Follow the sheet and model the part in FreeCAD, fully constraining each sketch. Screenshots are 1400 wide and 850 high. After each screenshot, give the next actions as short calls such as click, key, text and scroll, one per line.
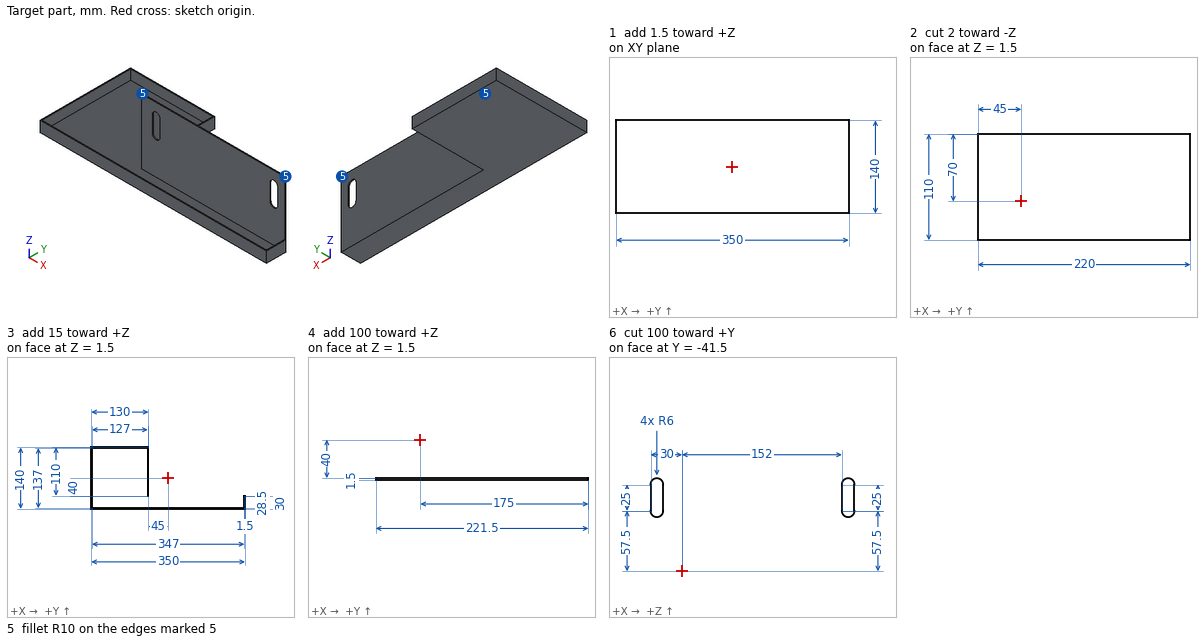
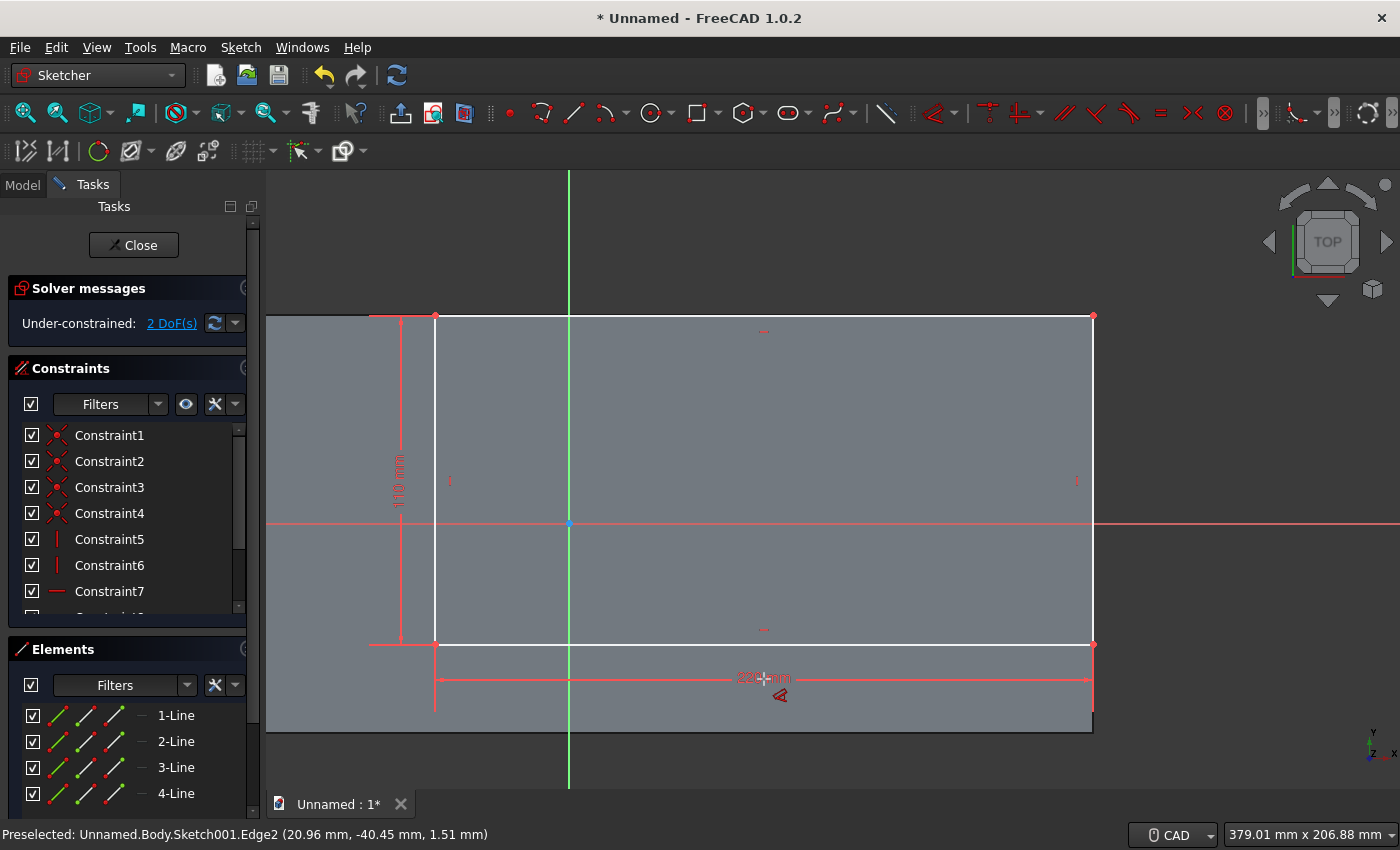
click(435, 316)
click(502, 282)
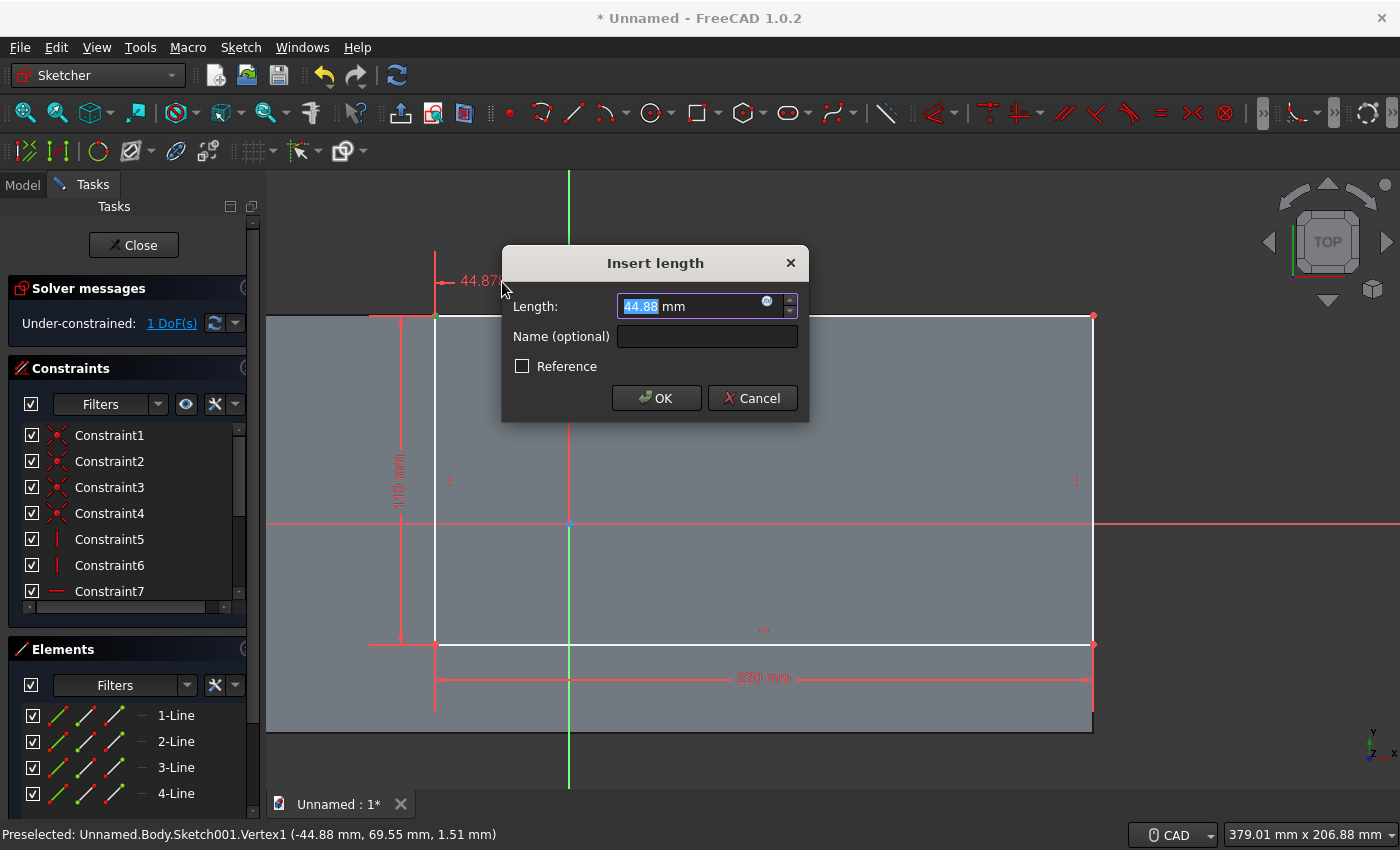
text(45)
key(Return)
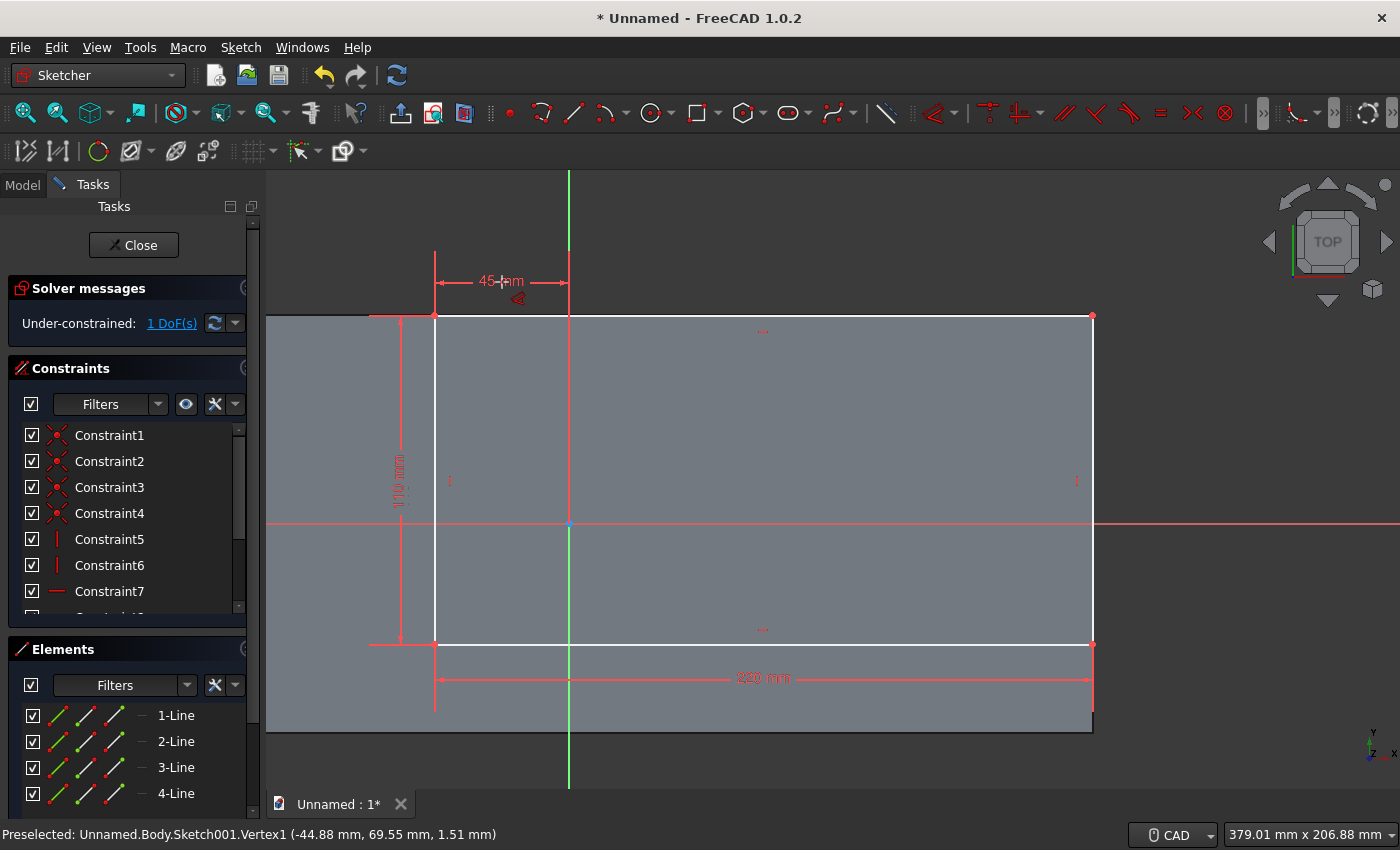
click(435, 316)
click(401, 420)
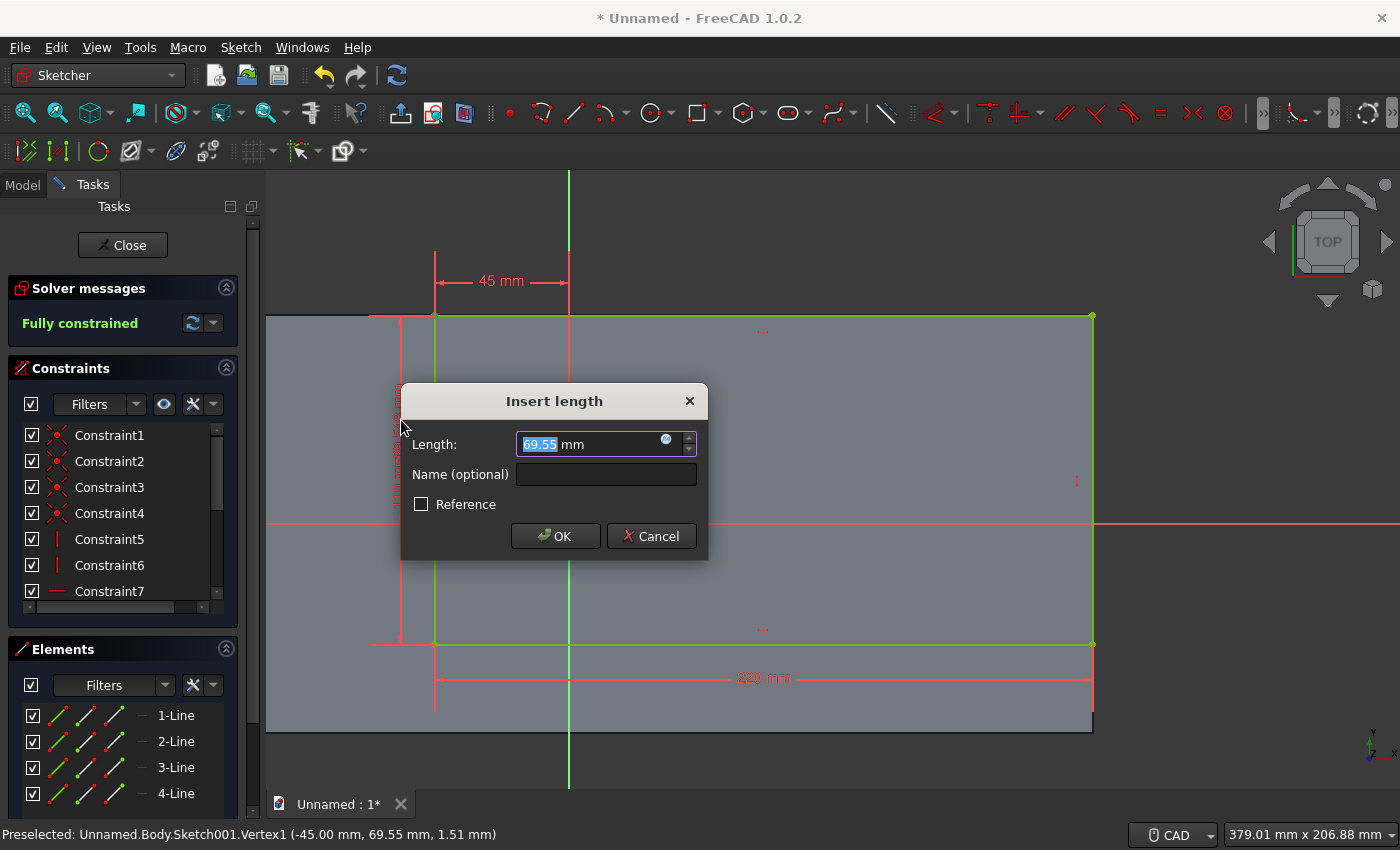
text(70)
key(Return)
key(Escape)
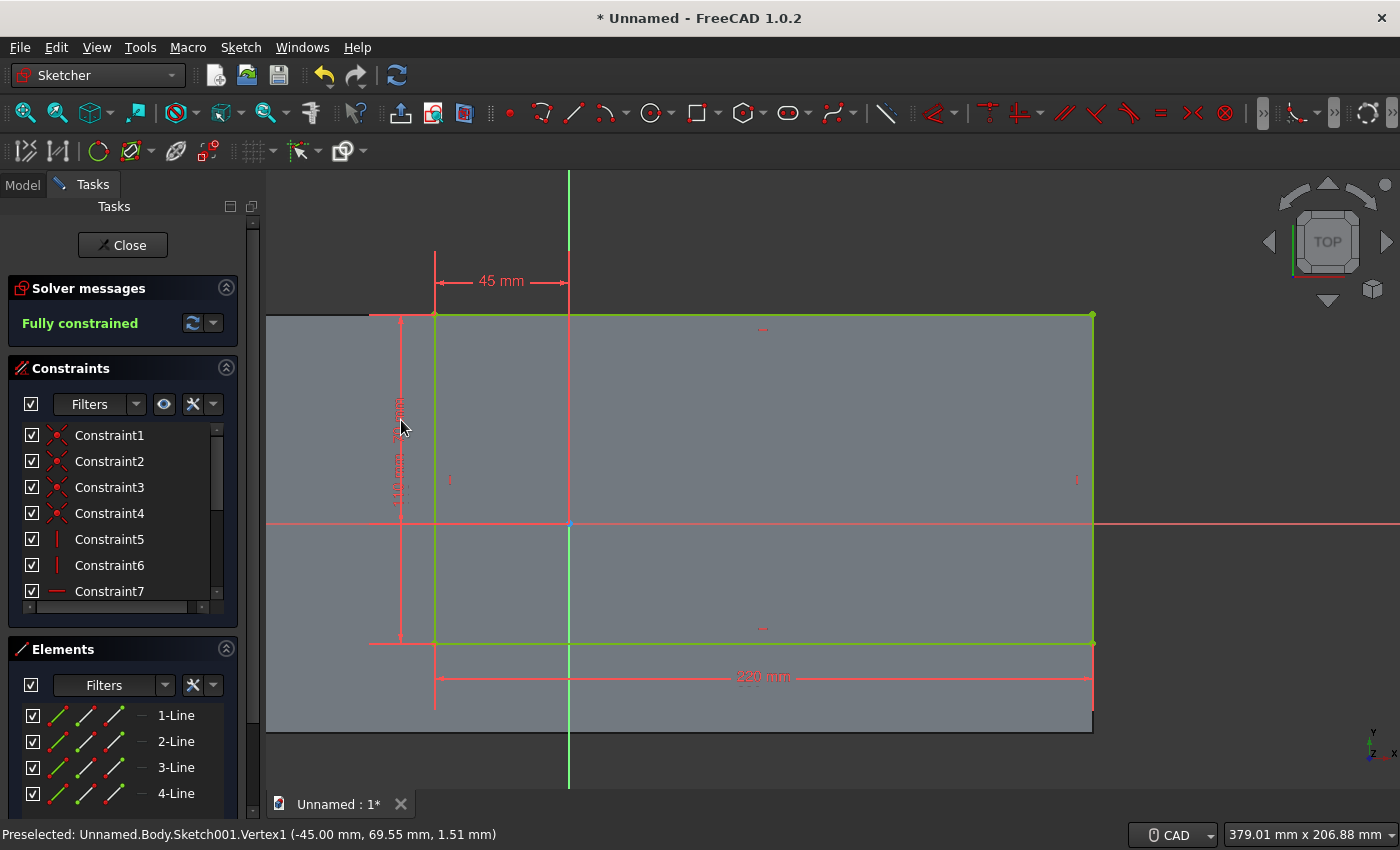
click(123, 245)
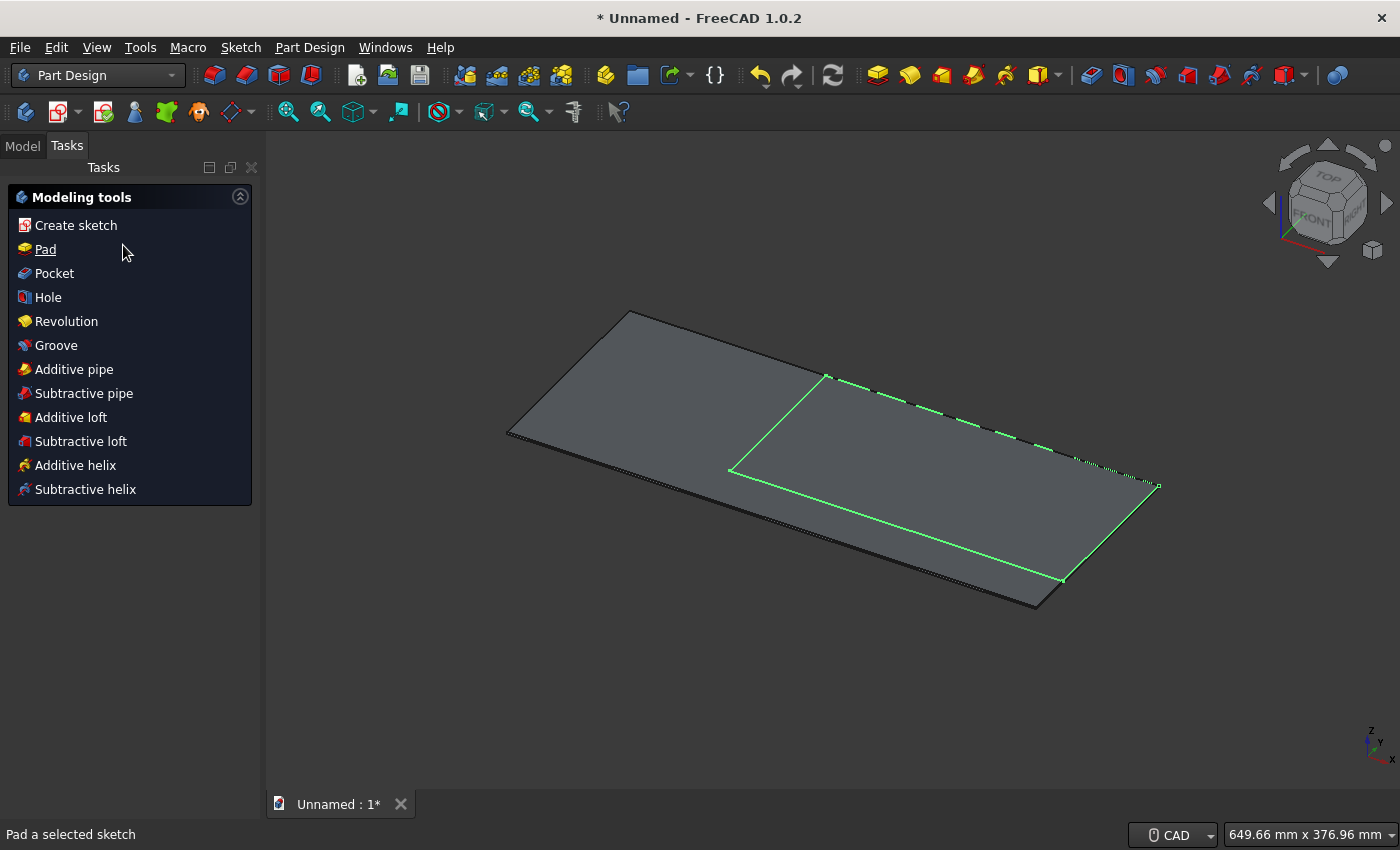
click(1092, 76)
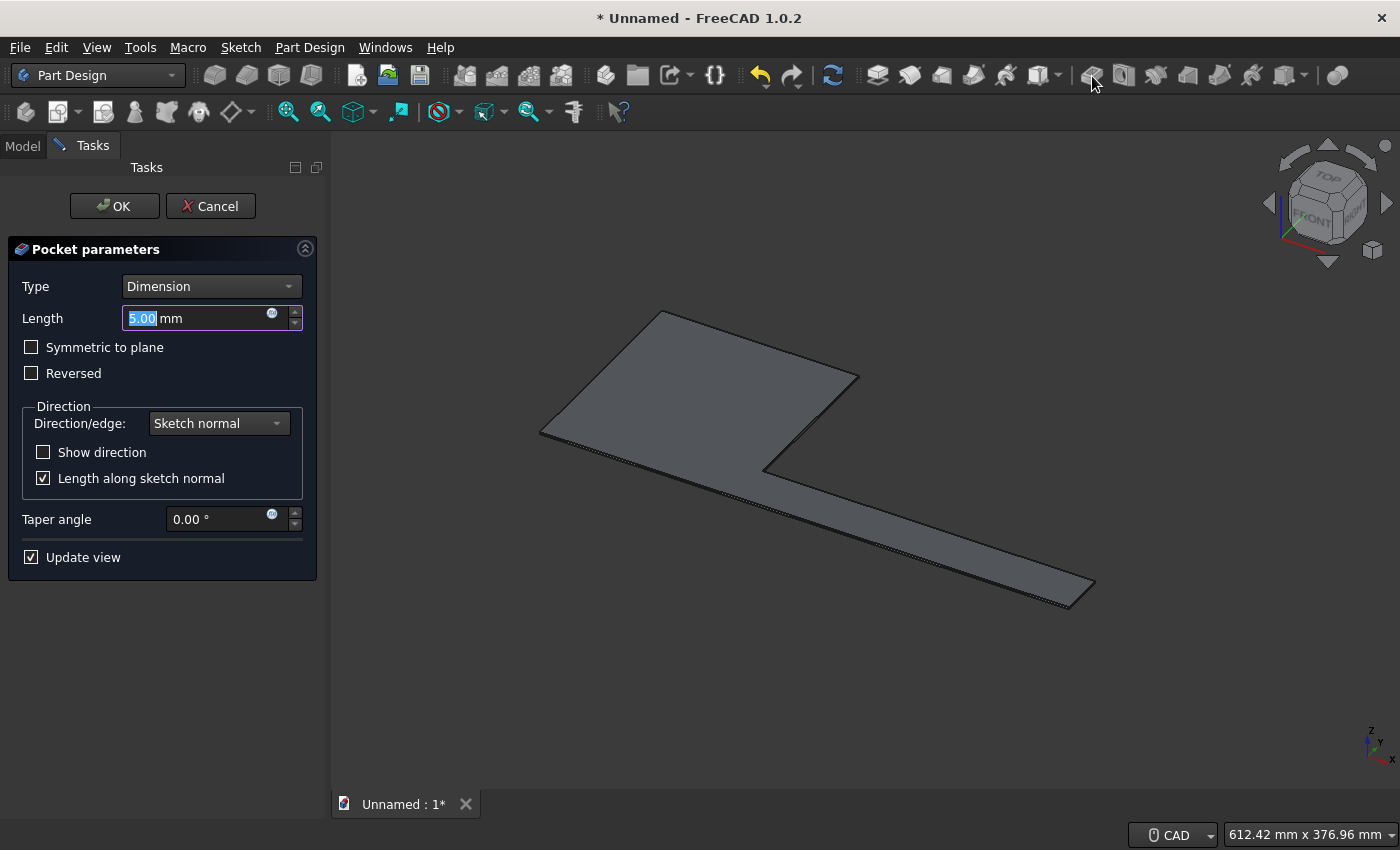
text(2)
key(Tab)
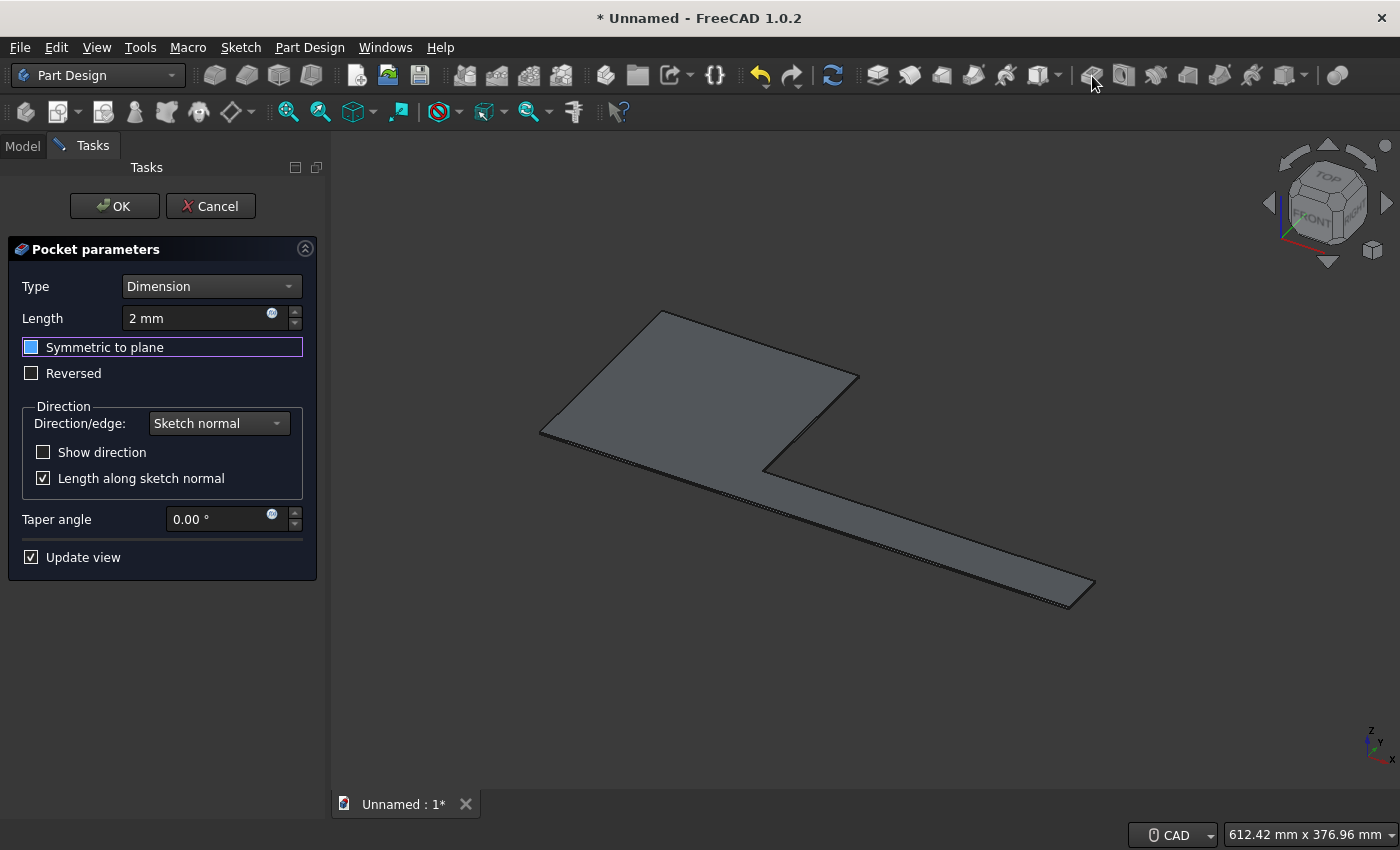
click(115, 206)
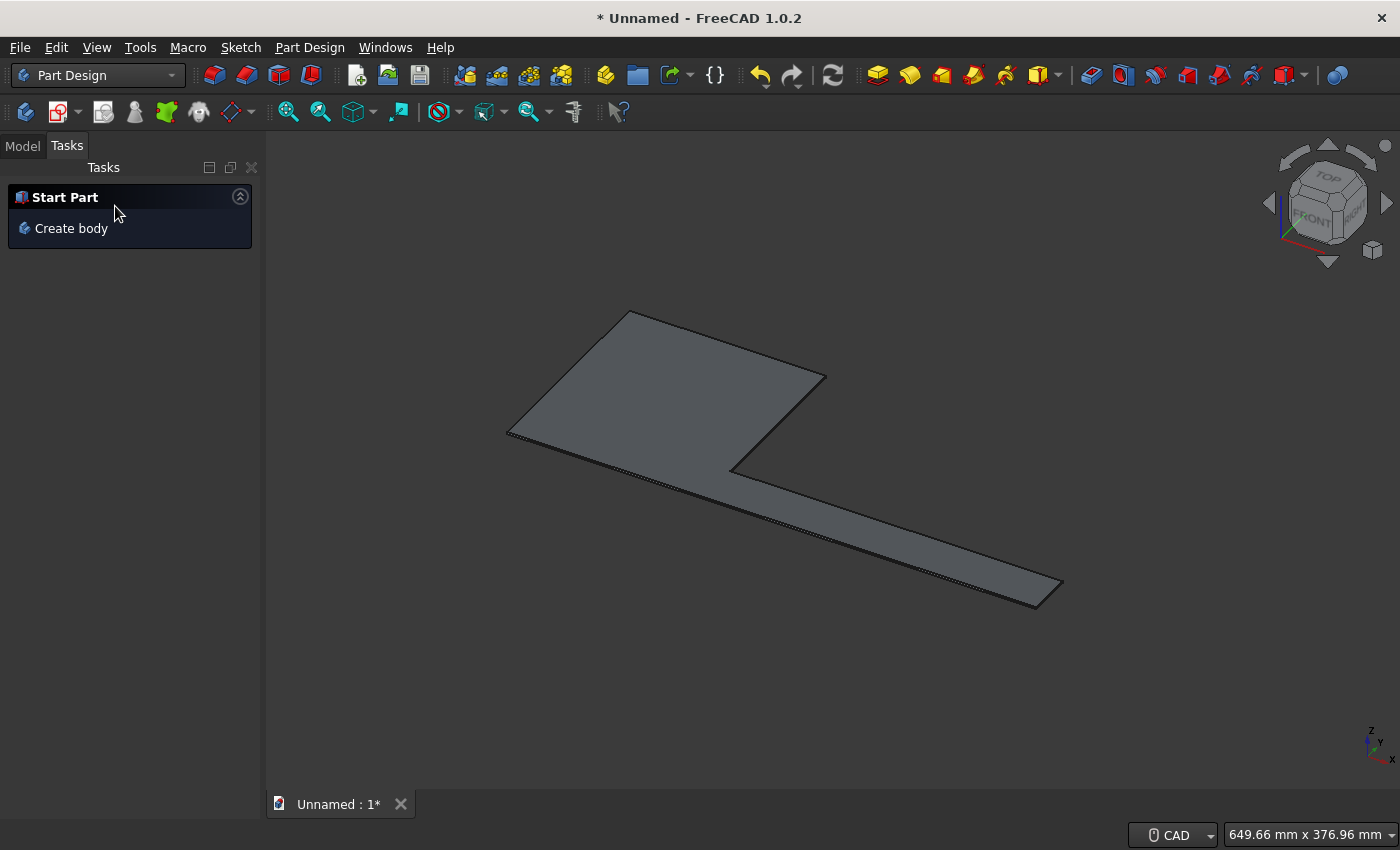
click(682, 408)